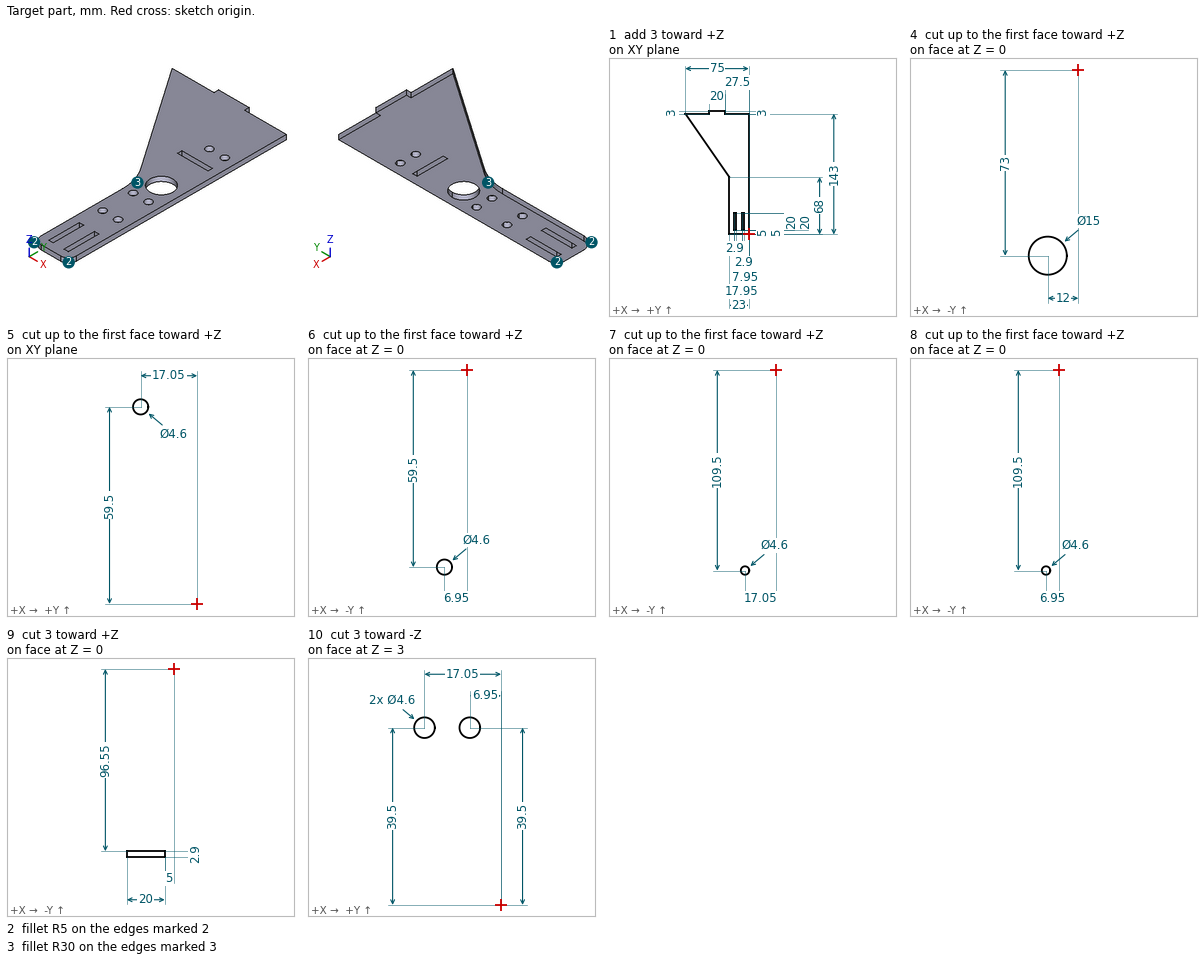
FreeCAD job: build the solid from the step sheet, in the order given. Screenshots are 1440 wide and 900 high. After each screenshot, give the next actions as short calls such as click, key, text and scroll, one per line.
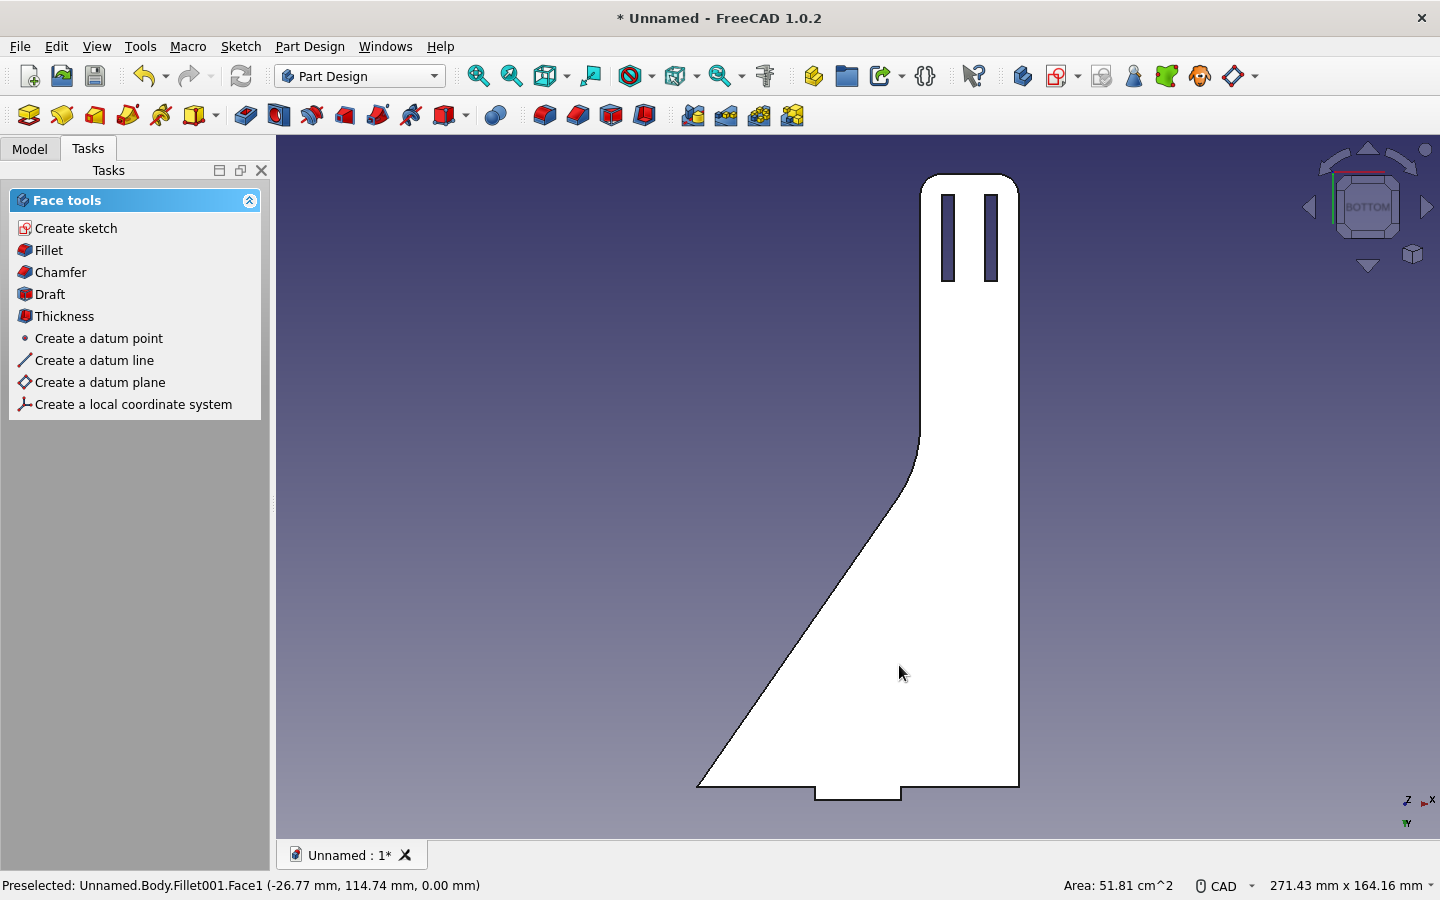
click(1056, 76)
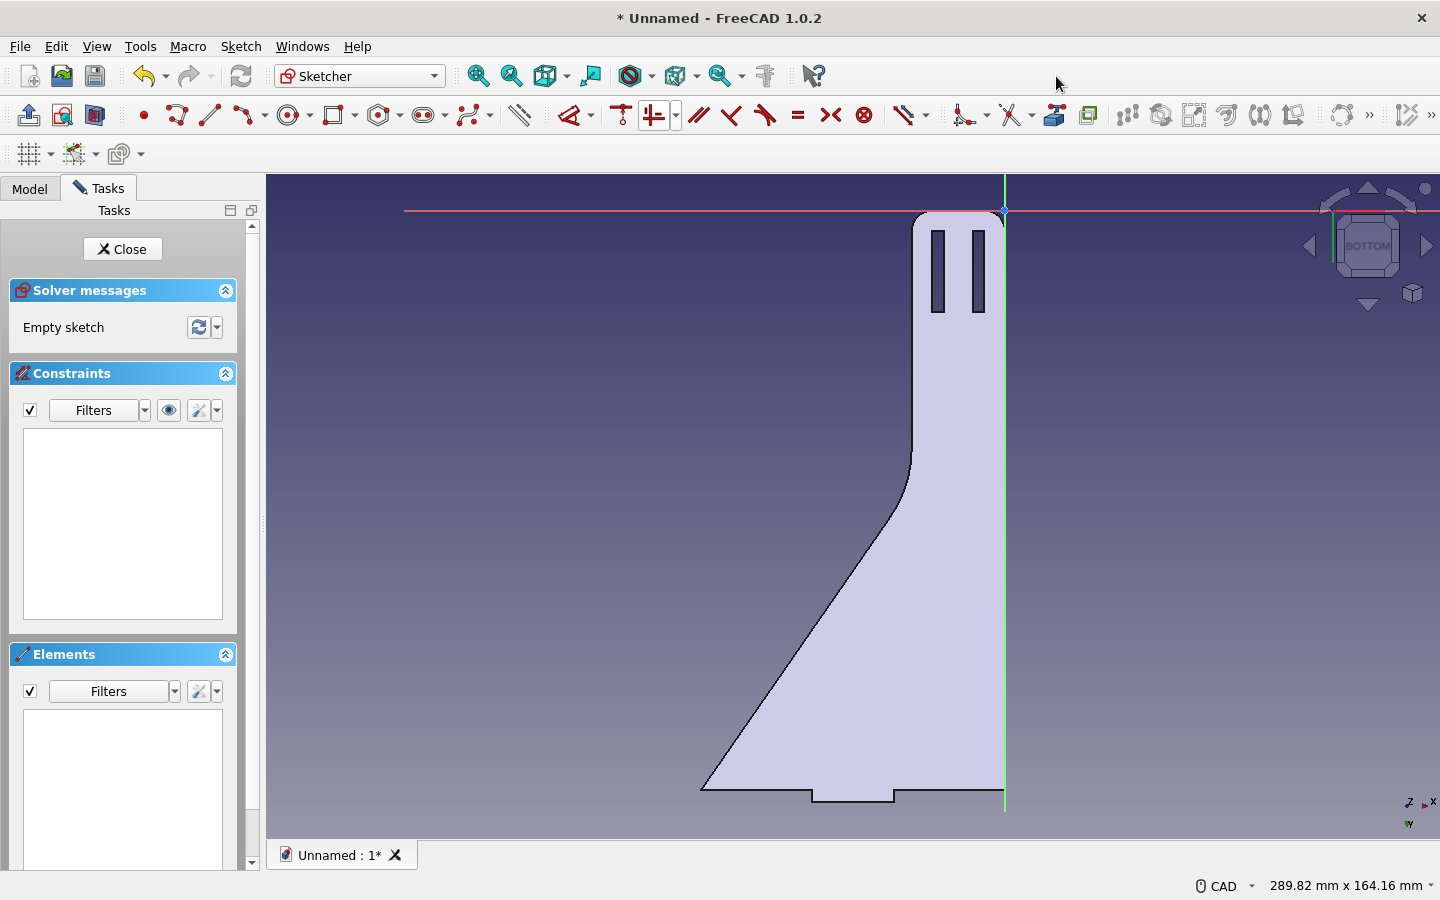
scroll(983, 506, up, 10)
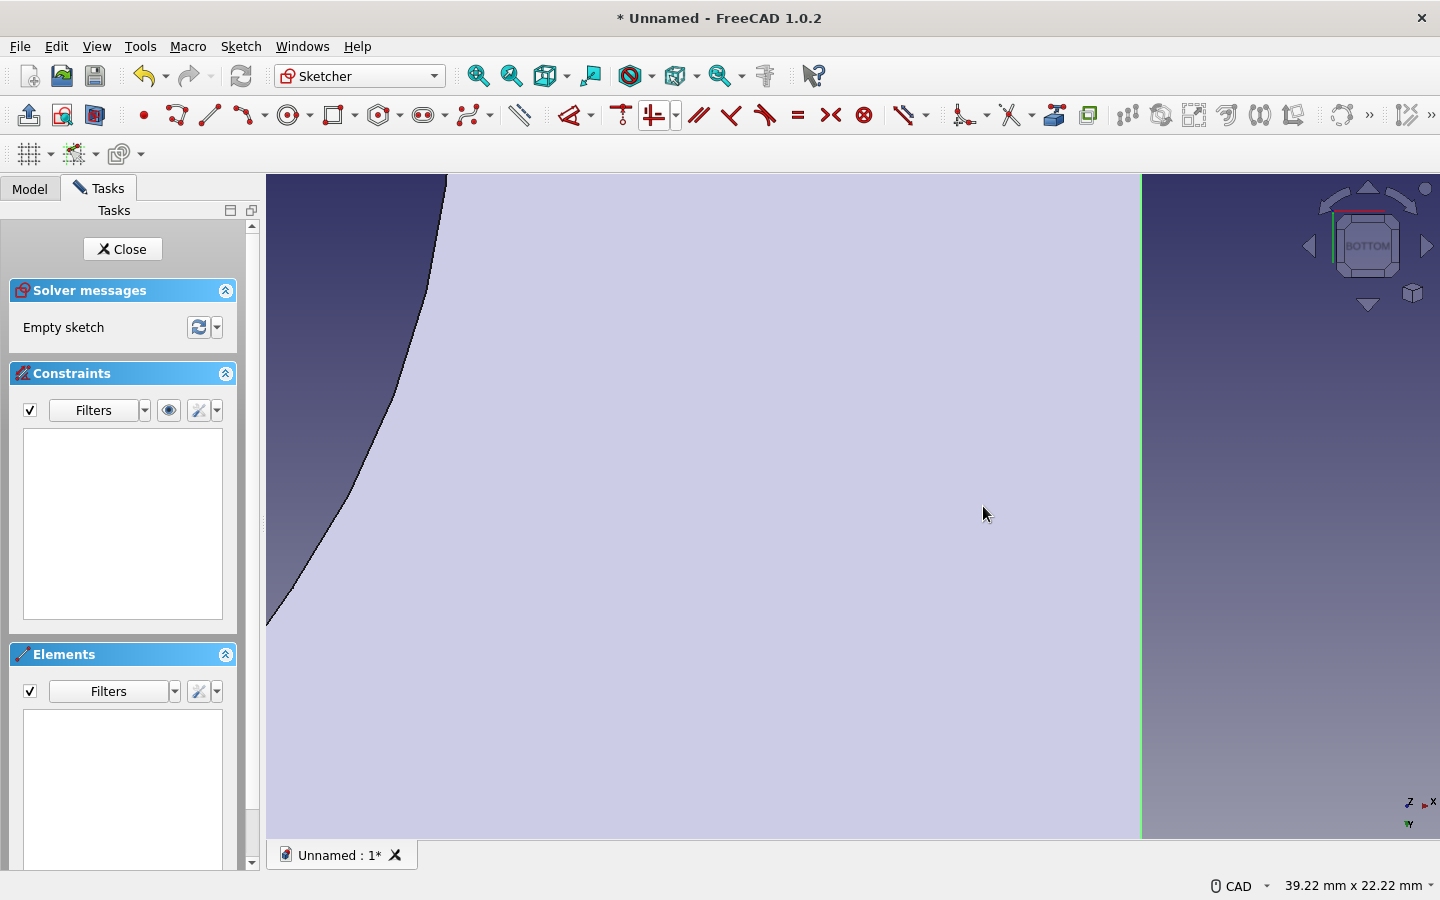
key(g)
key(c)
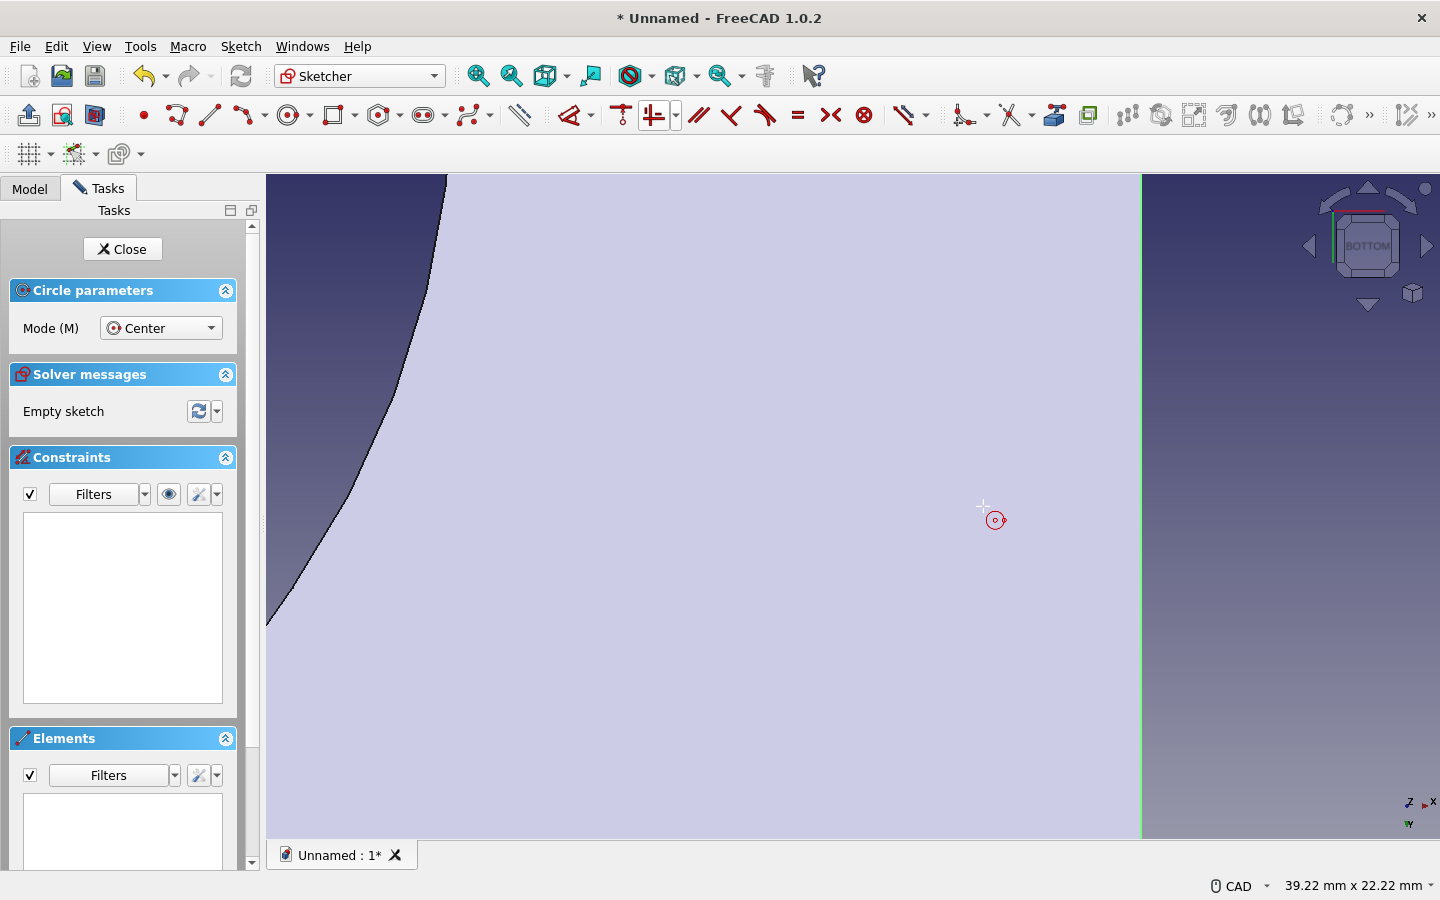
click(782, 506)
move(941, 348)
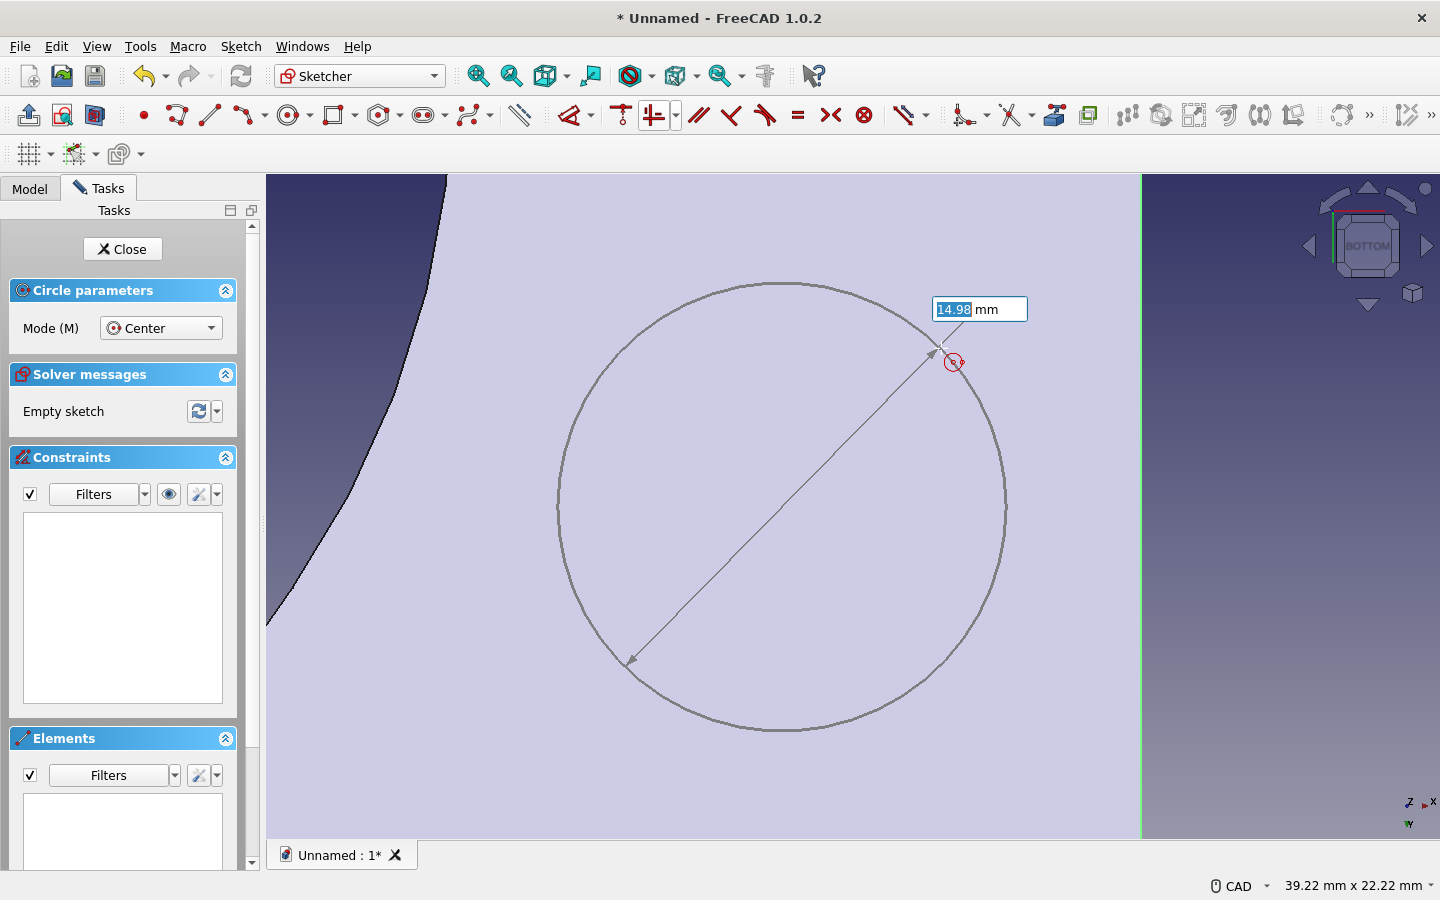
text(15)
key(Return)
key(Escape)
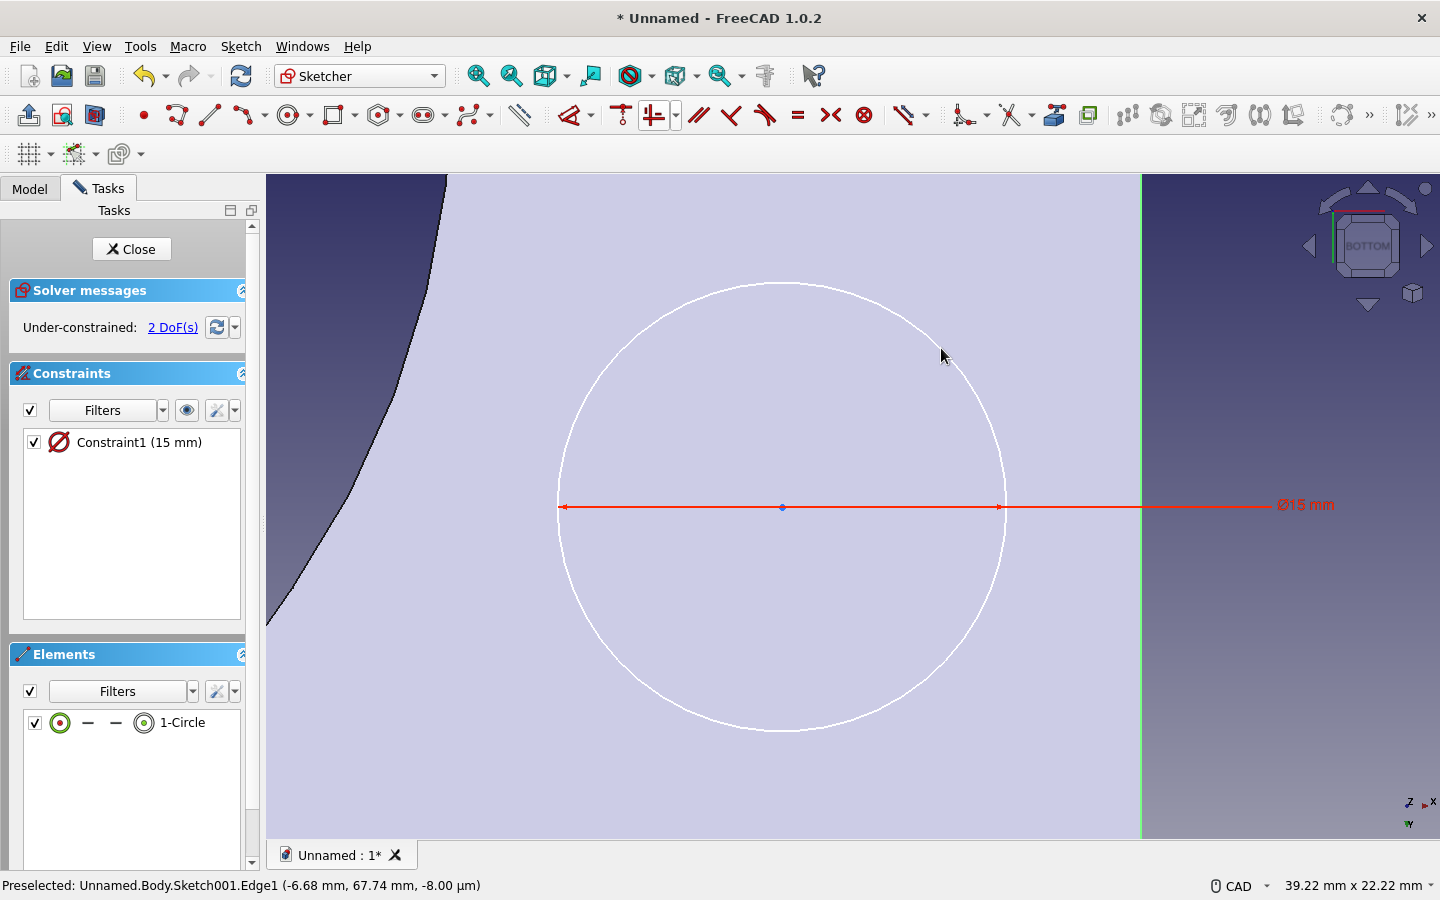
click(568, 116)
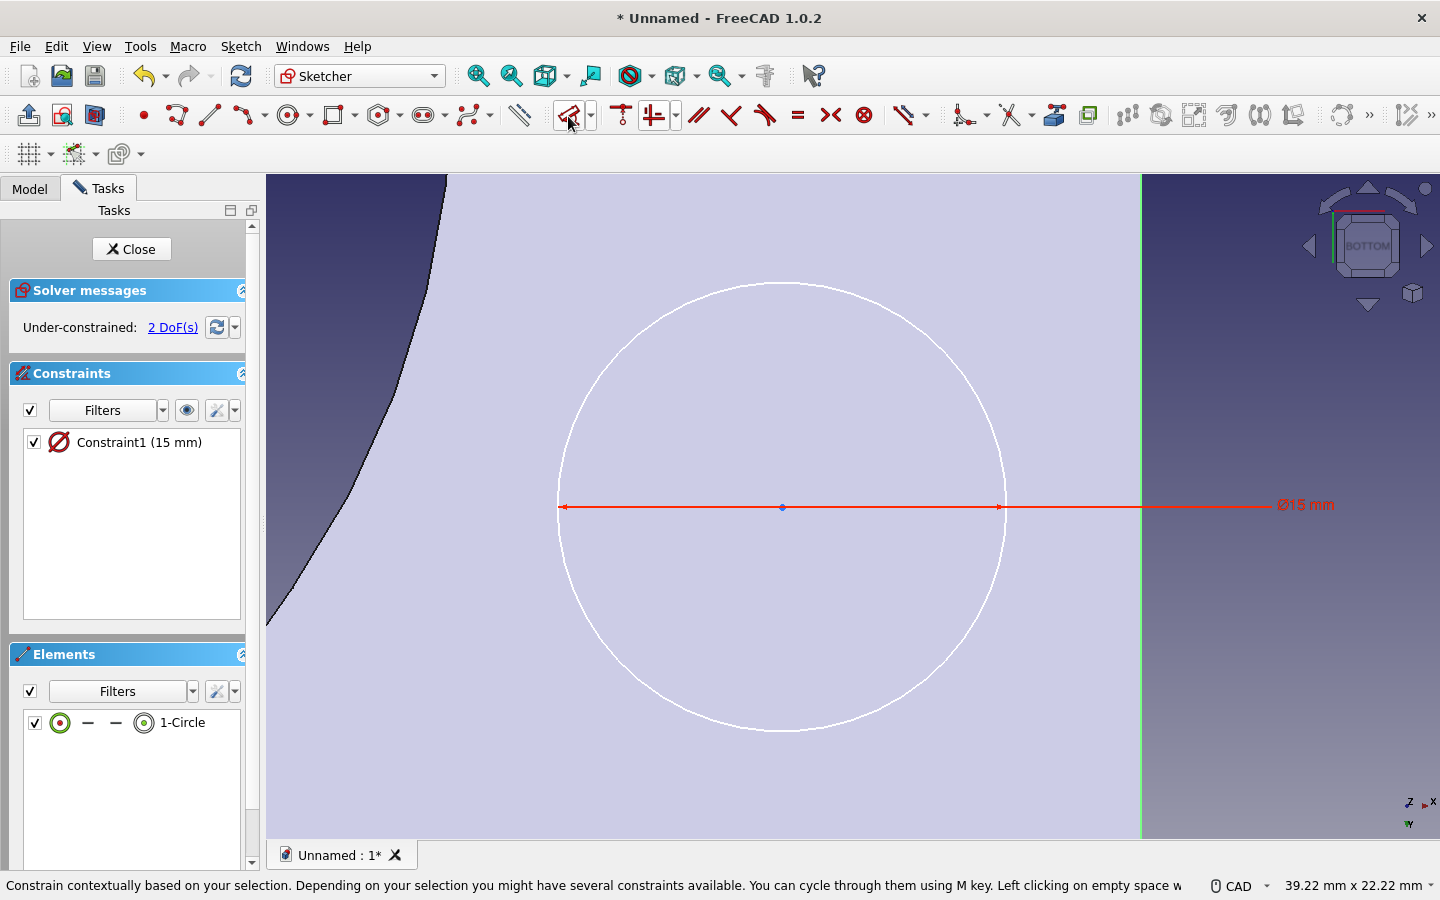
click(782, 507)
click(961, 541)